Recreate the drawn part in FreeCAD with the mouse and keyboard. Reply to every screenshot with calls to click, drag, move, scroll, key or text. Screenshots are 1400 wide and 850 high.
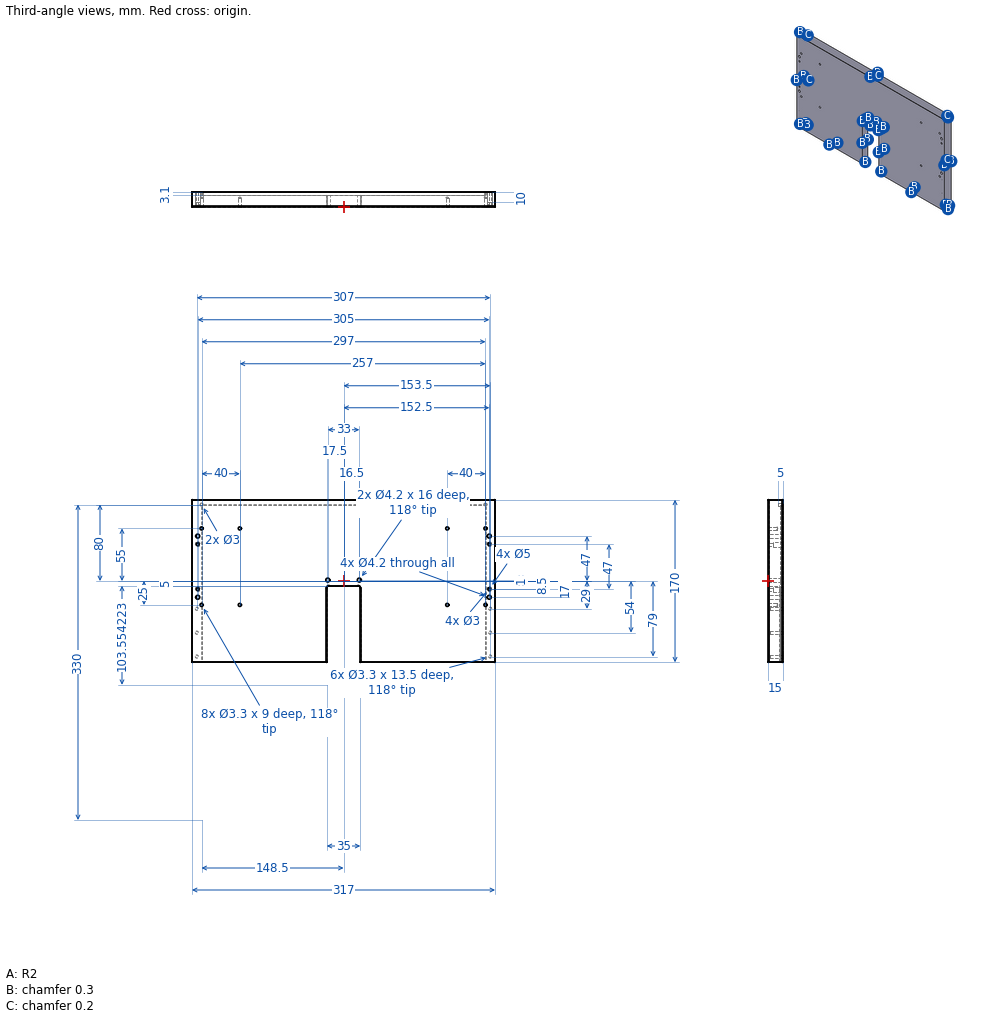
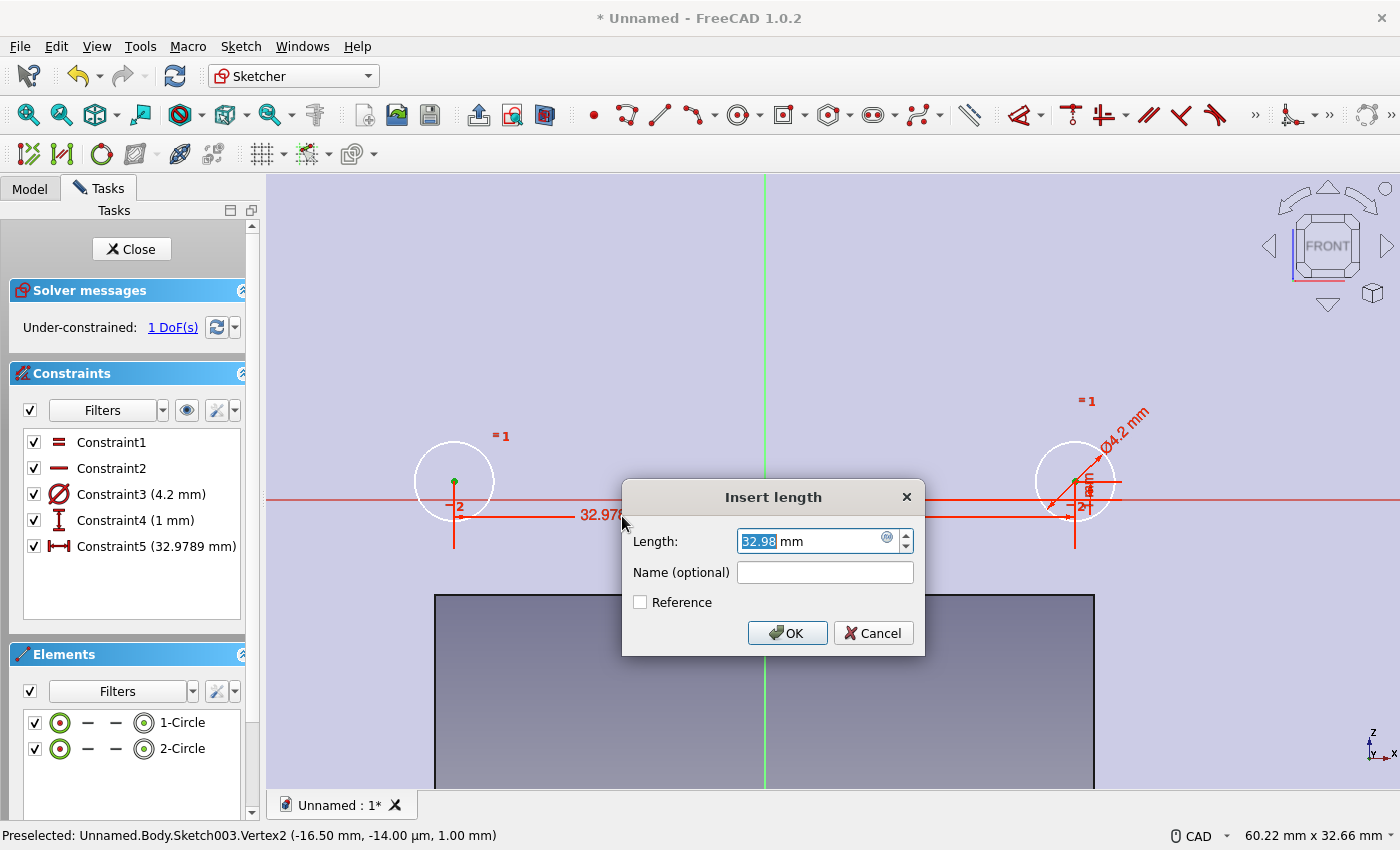
text(33)
key(Return)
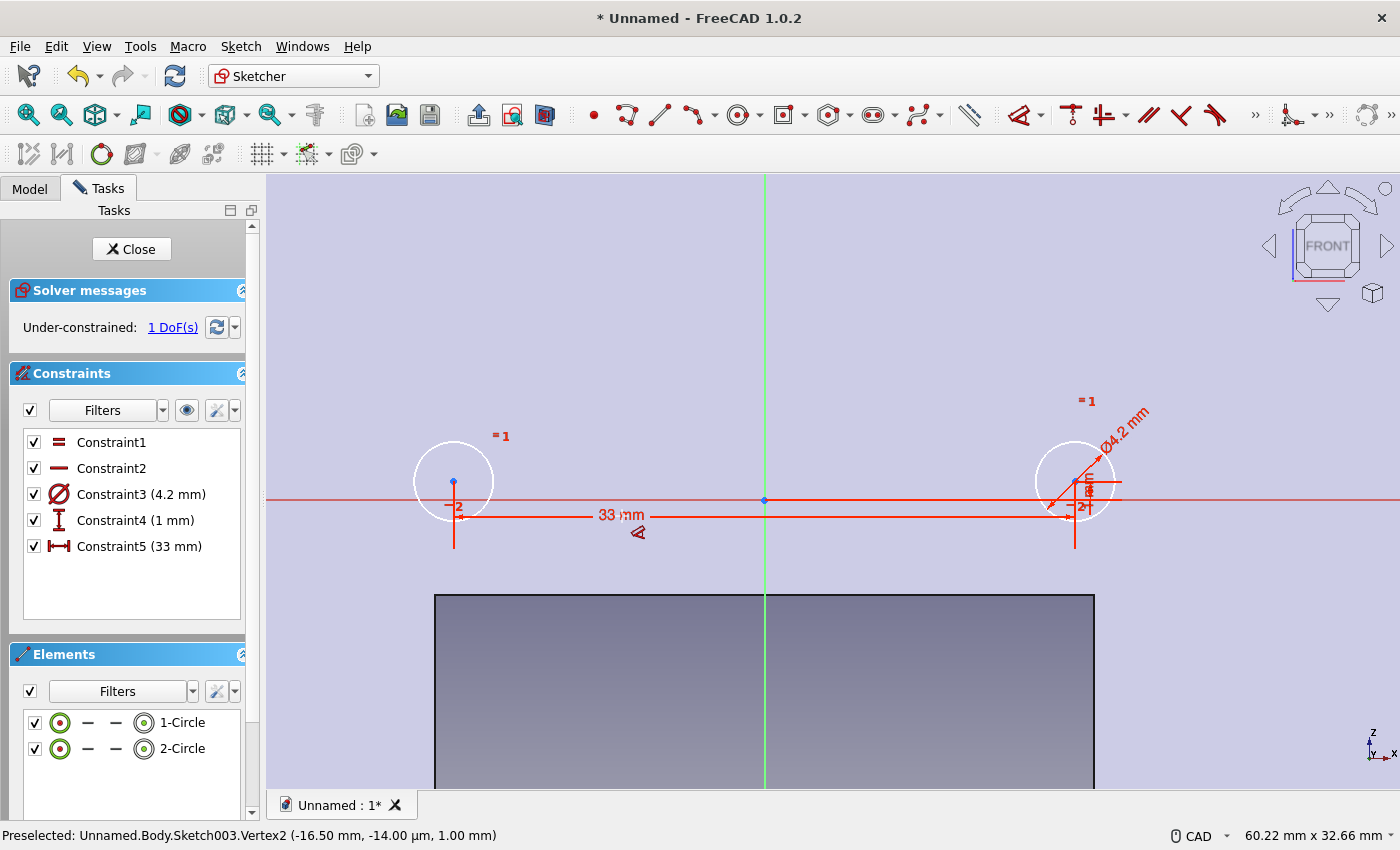
click(1075, 482)
click(920, 534)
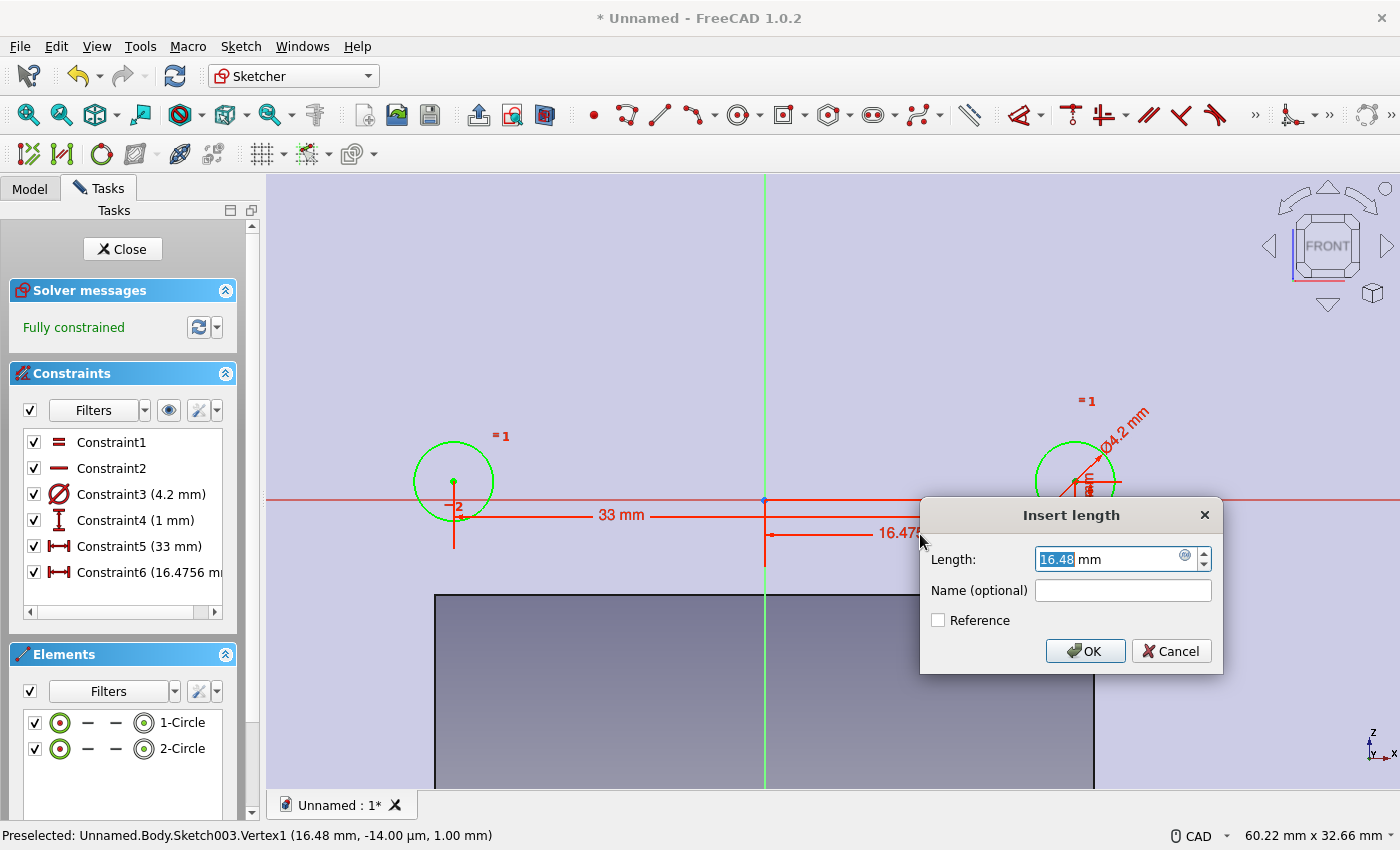
text(16.5)
key(Return)
key(Escape)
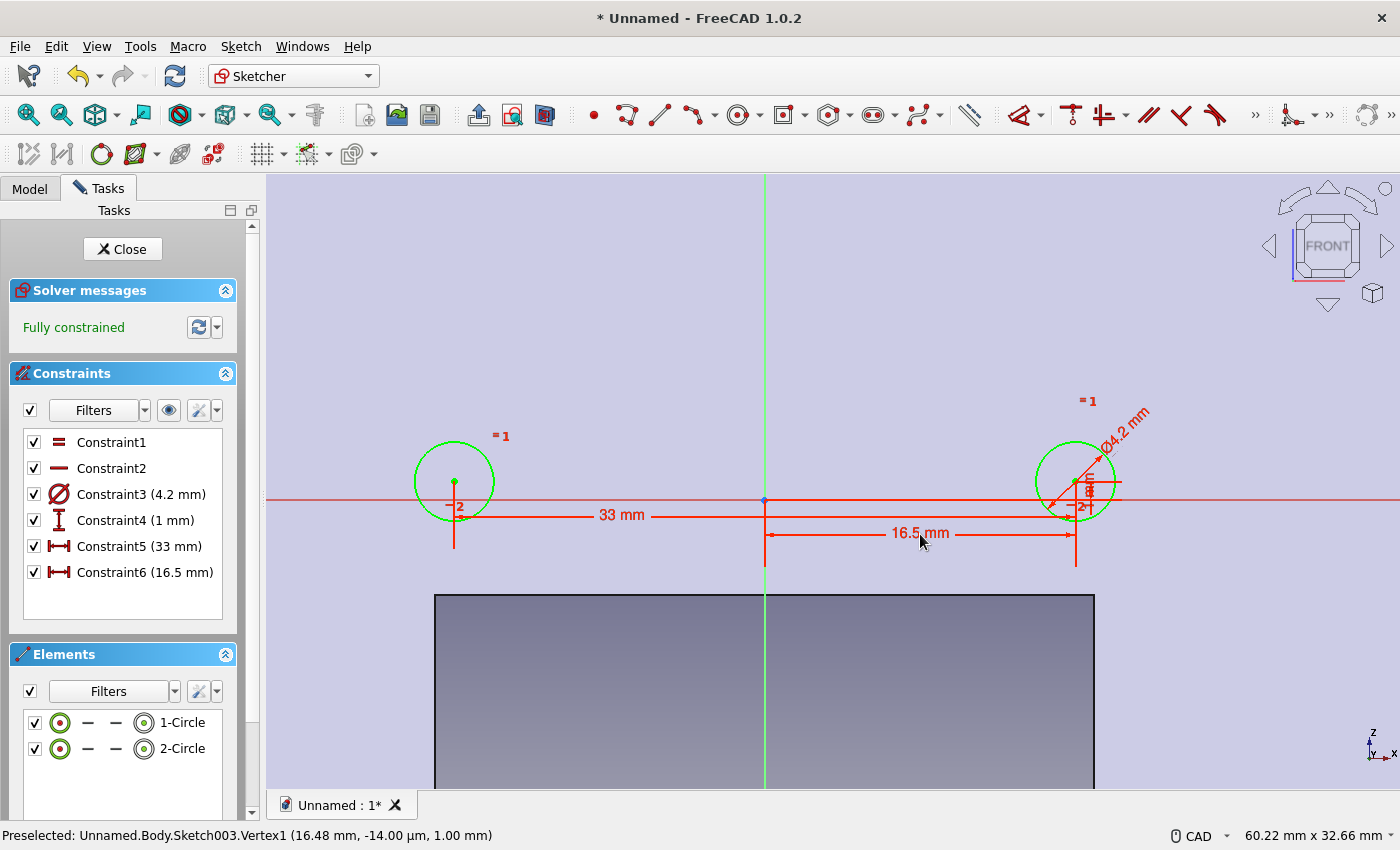
click(123, 249)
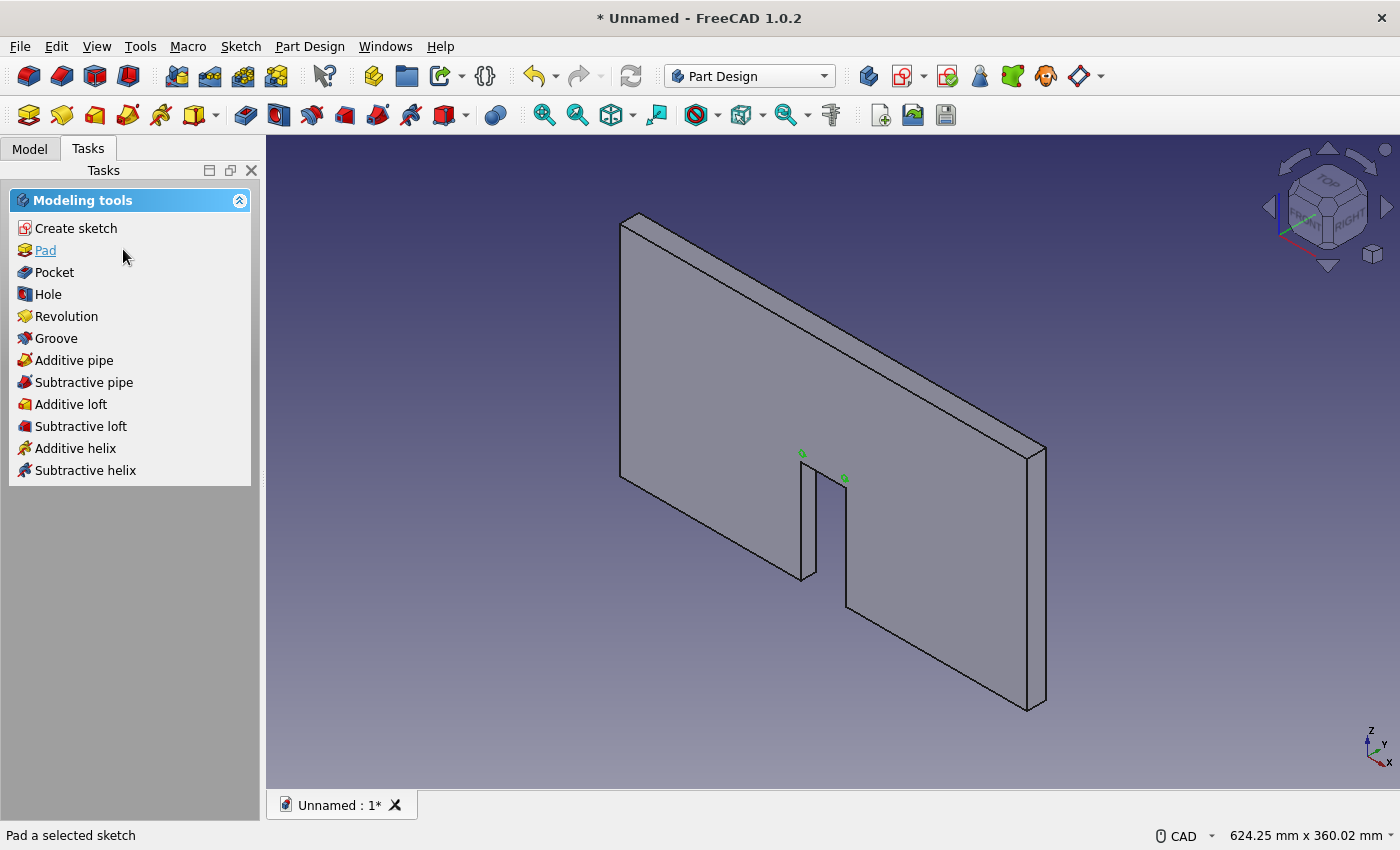
click(279, 116)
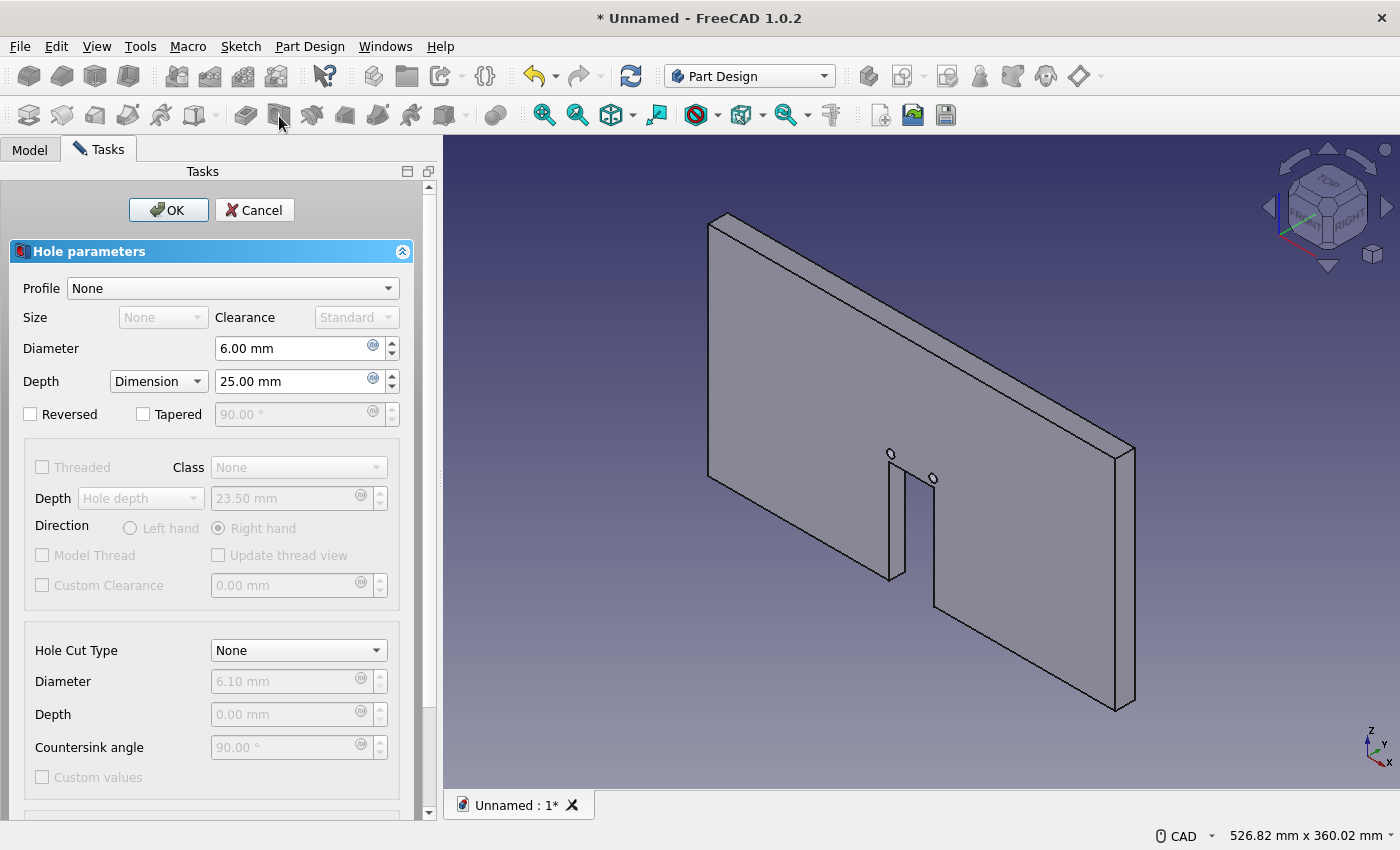
triple_click(300, 348)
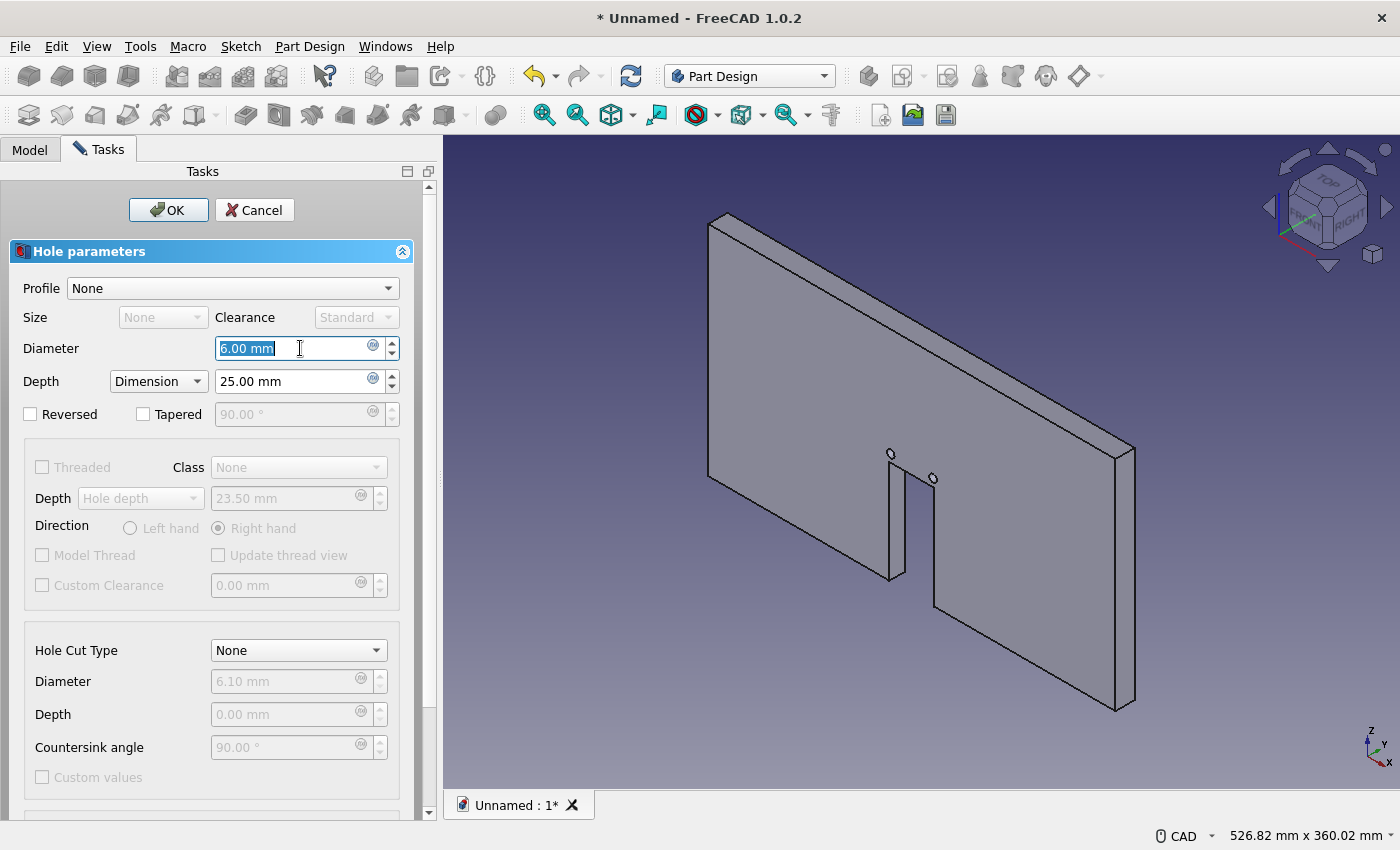
text(4.2)
key(Tab)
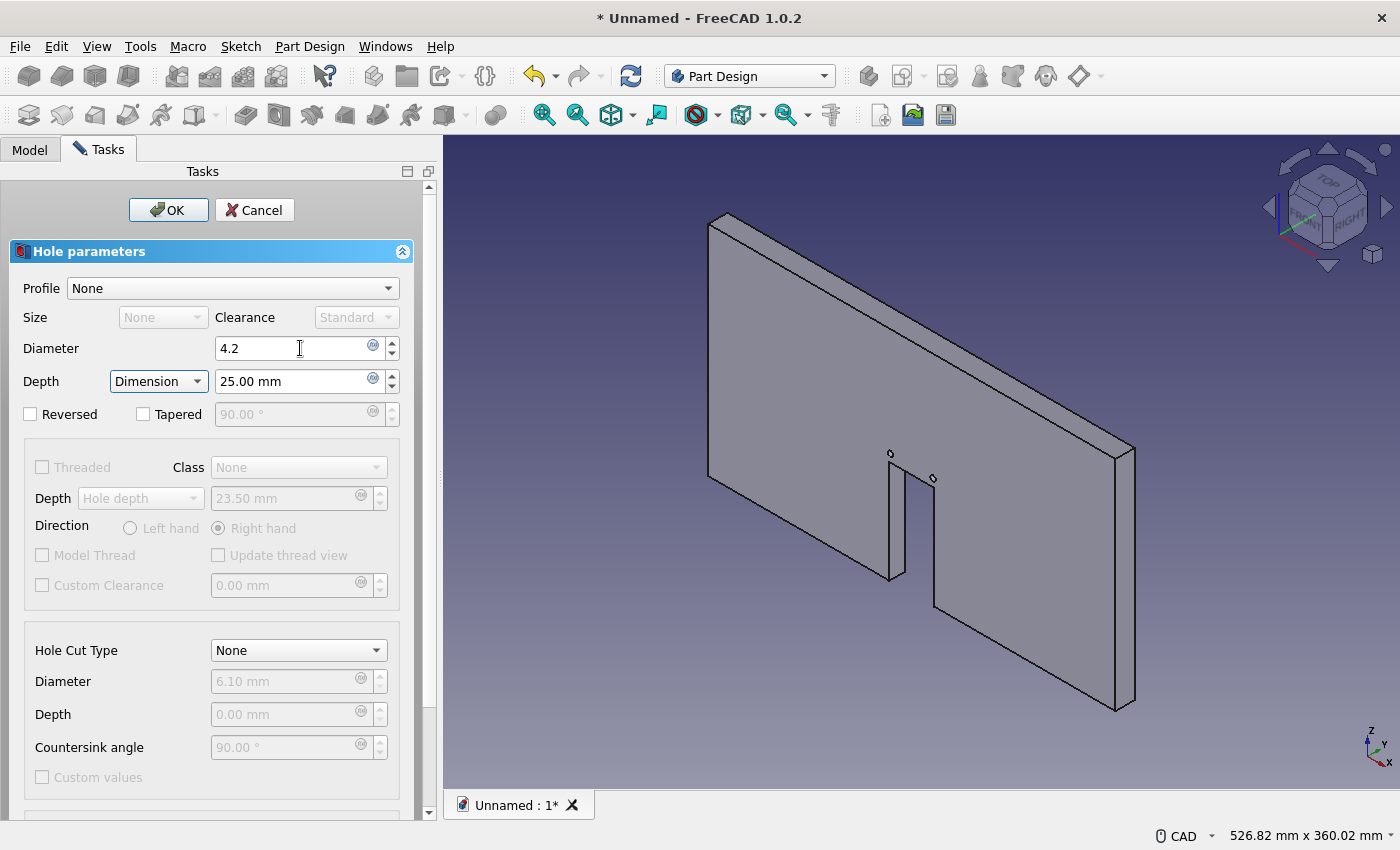
triple_click(300, 382)